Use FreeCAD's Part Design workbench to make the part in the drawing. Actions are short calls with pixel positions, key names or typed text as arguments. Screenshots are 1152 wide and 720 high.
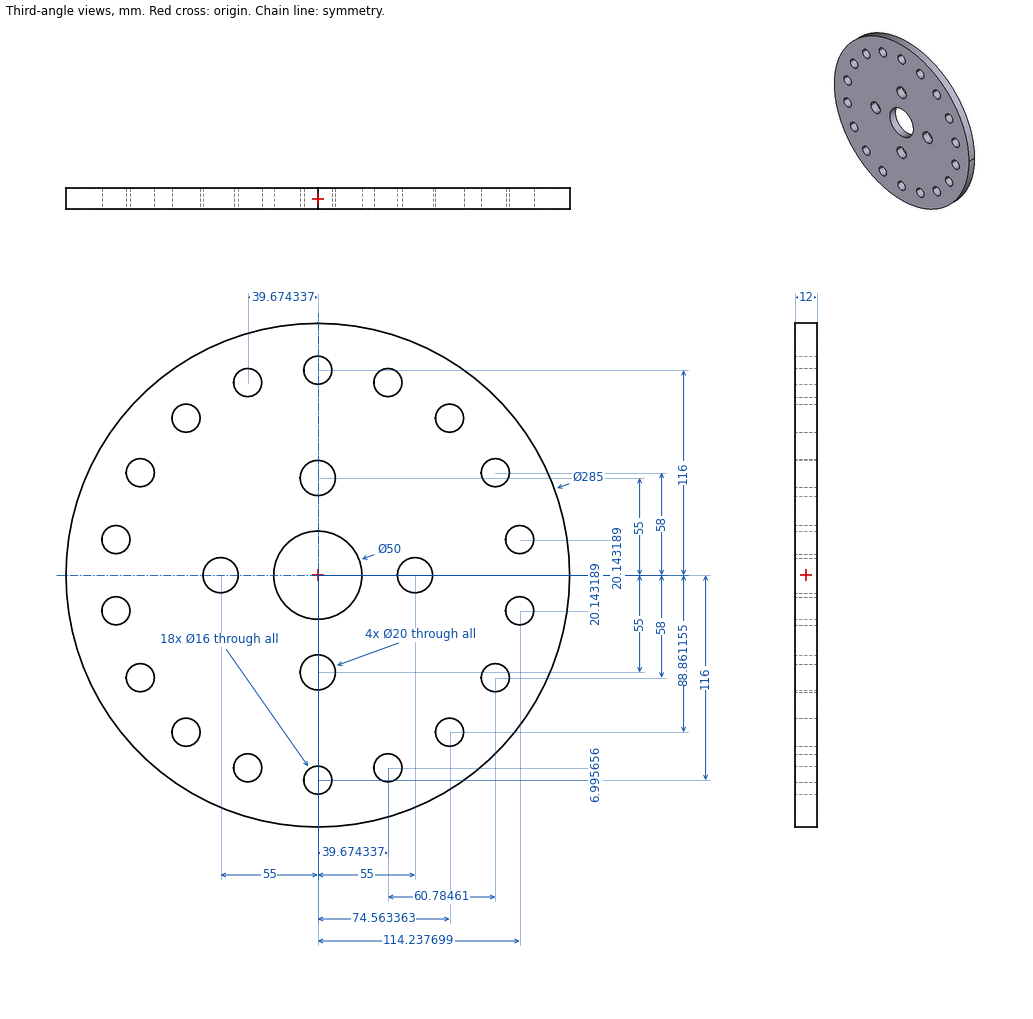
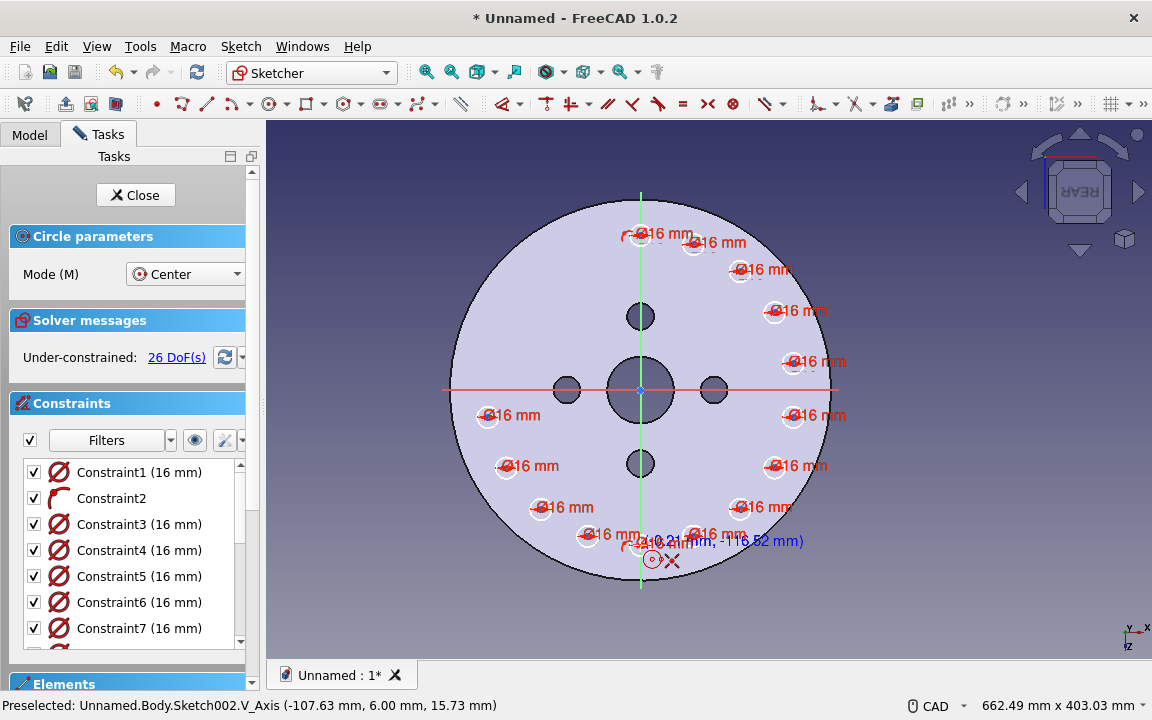
scroll(488, 363, up, 4)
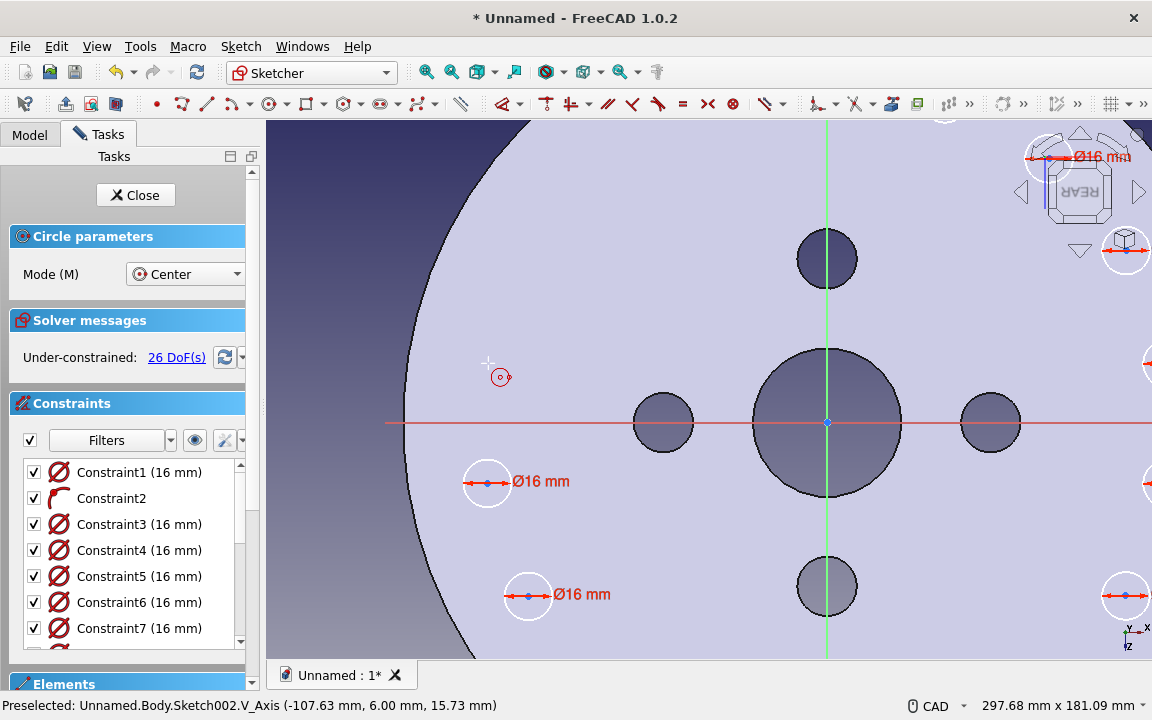
click(487, 363)
move(504, 346)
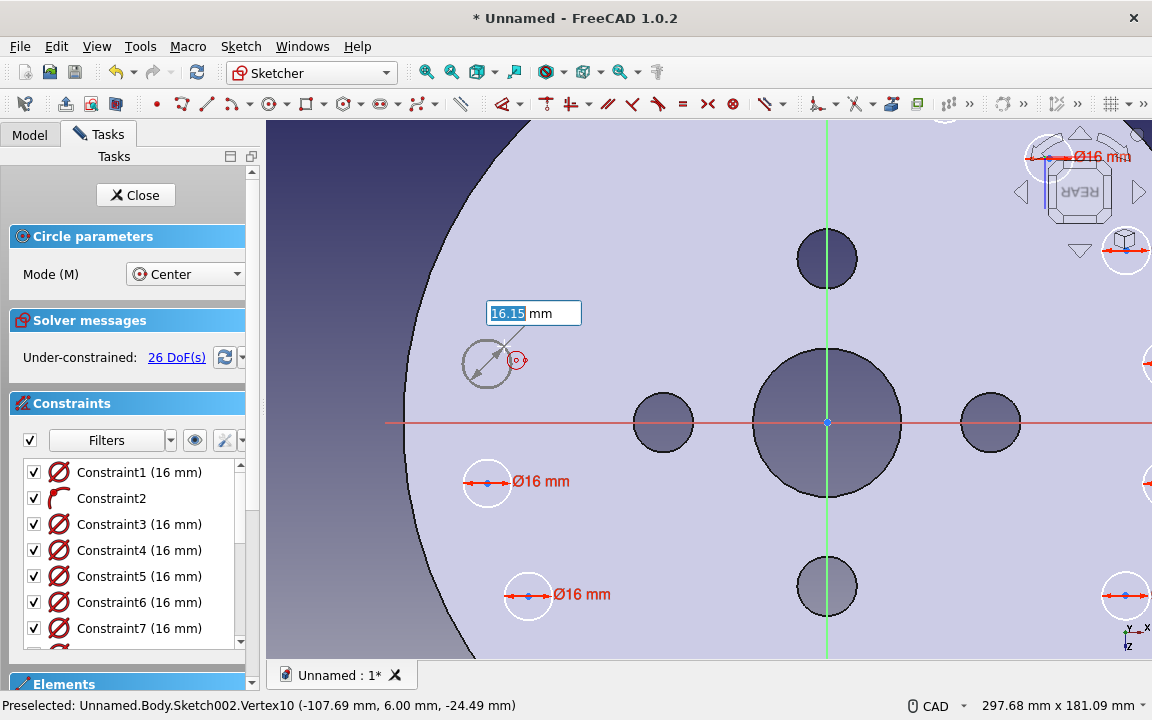
text(16)
key(Return)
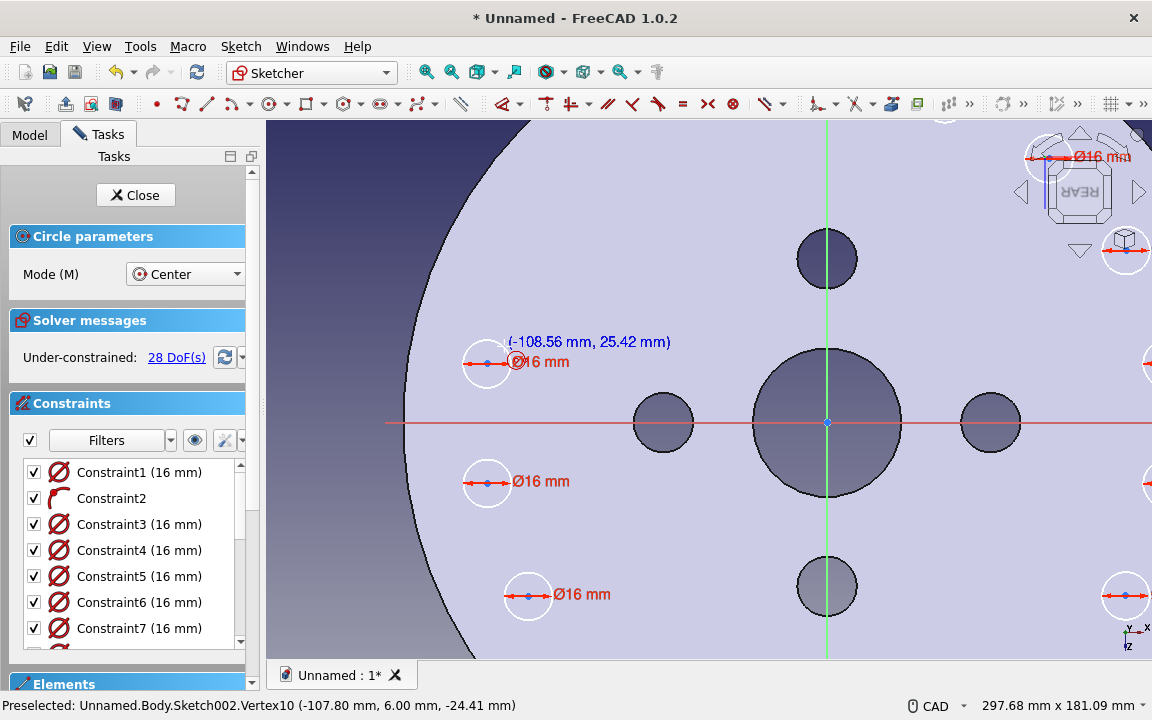
click(528, 250)
move(545, 233)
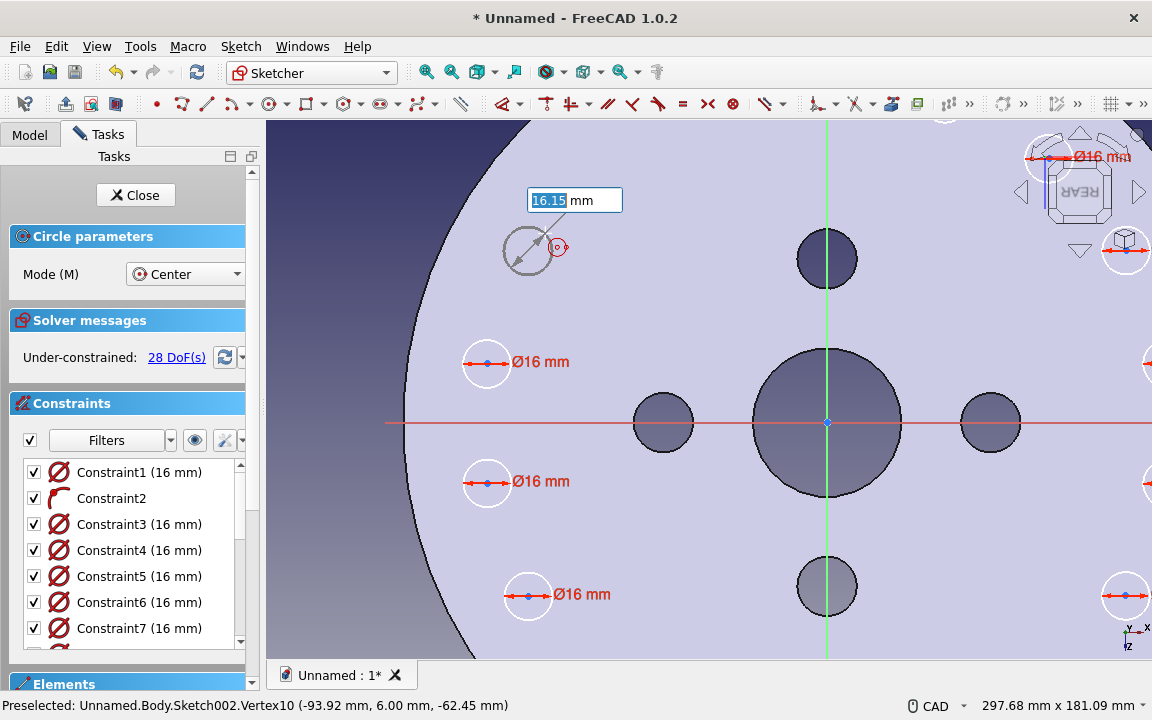
text(16)
key(Return)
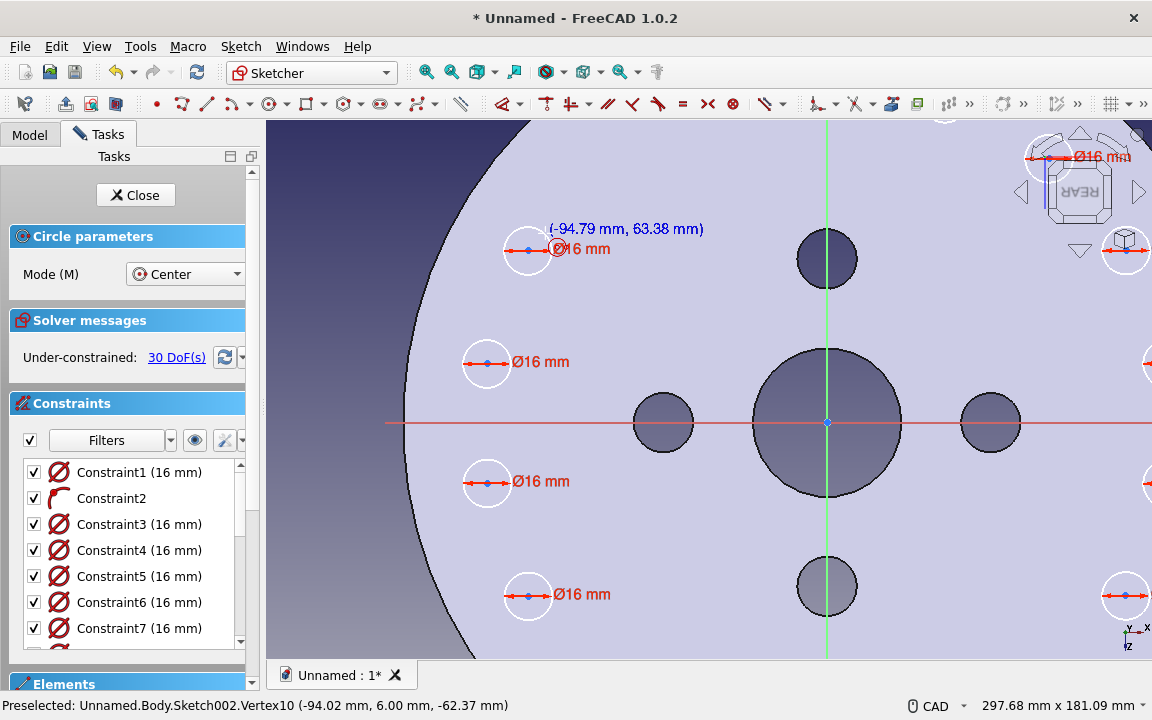
click(605, 158)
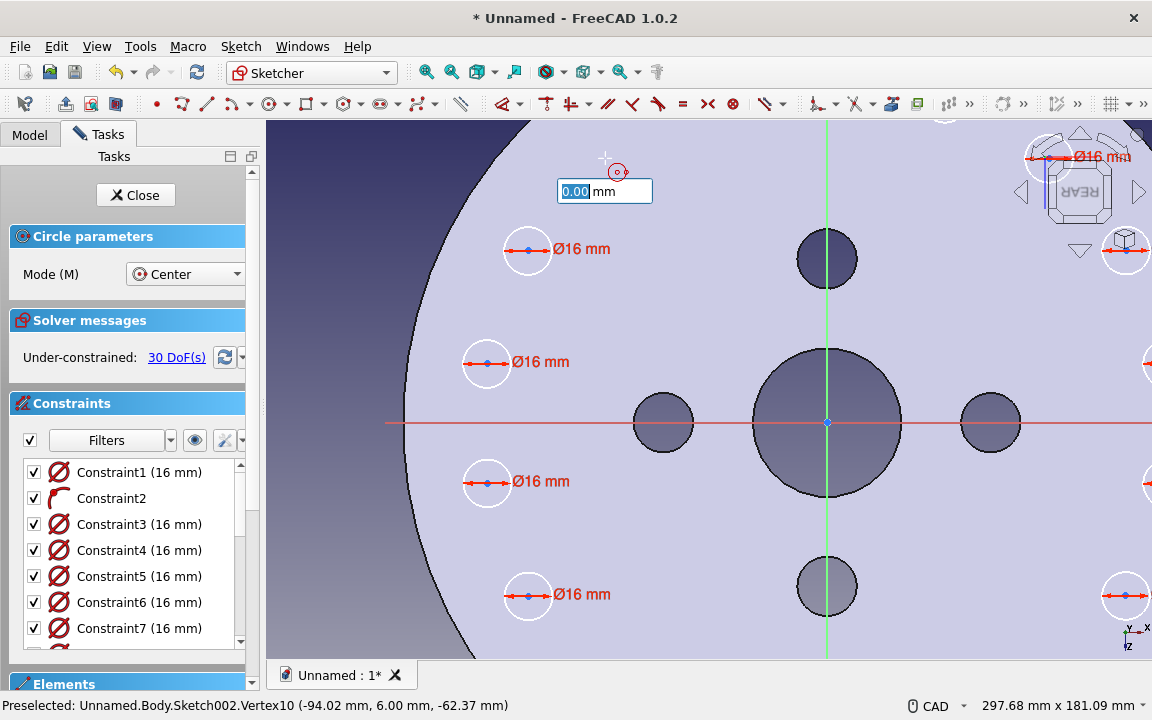
scroll(488, 362, down, 4)
move(548, 263)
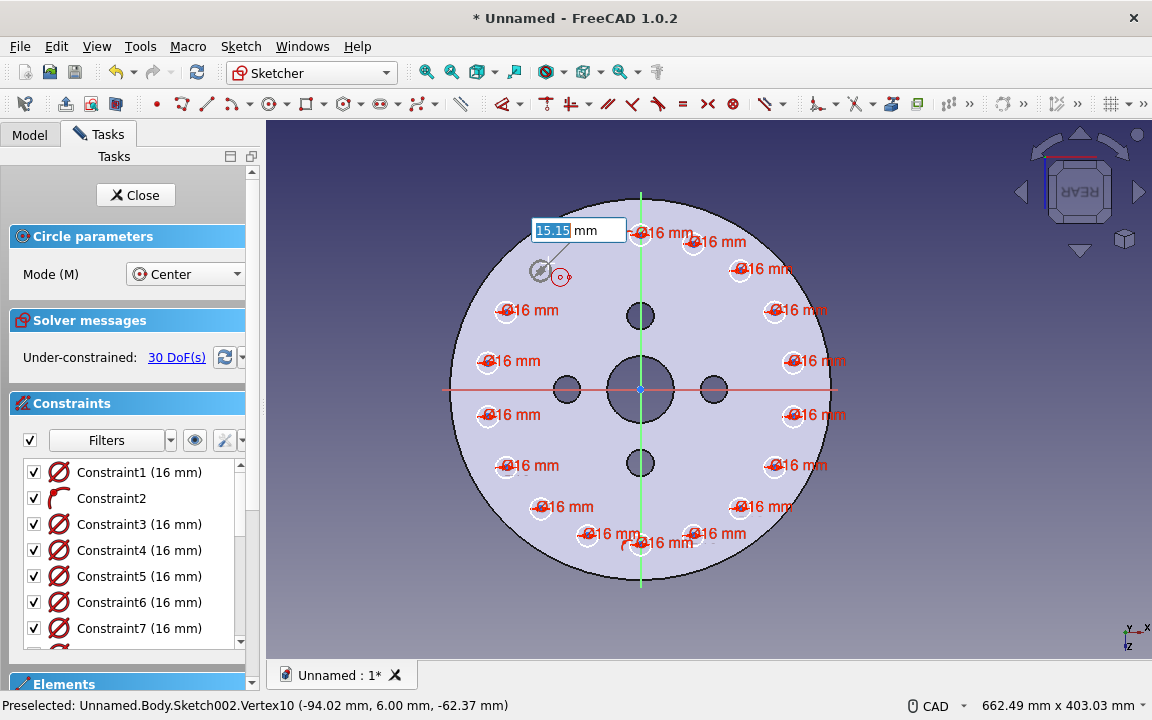
text(16)
key(Return)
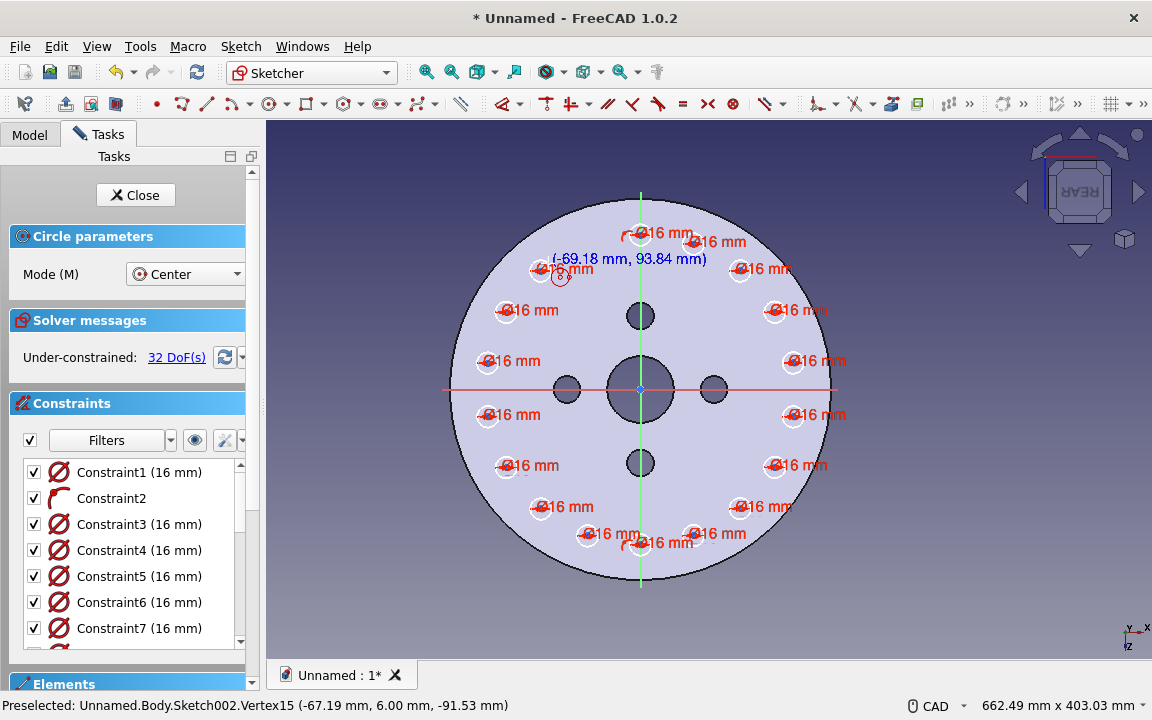
scroll(587, 244, up, 4)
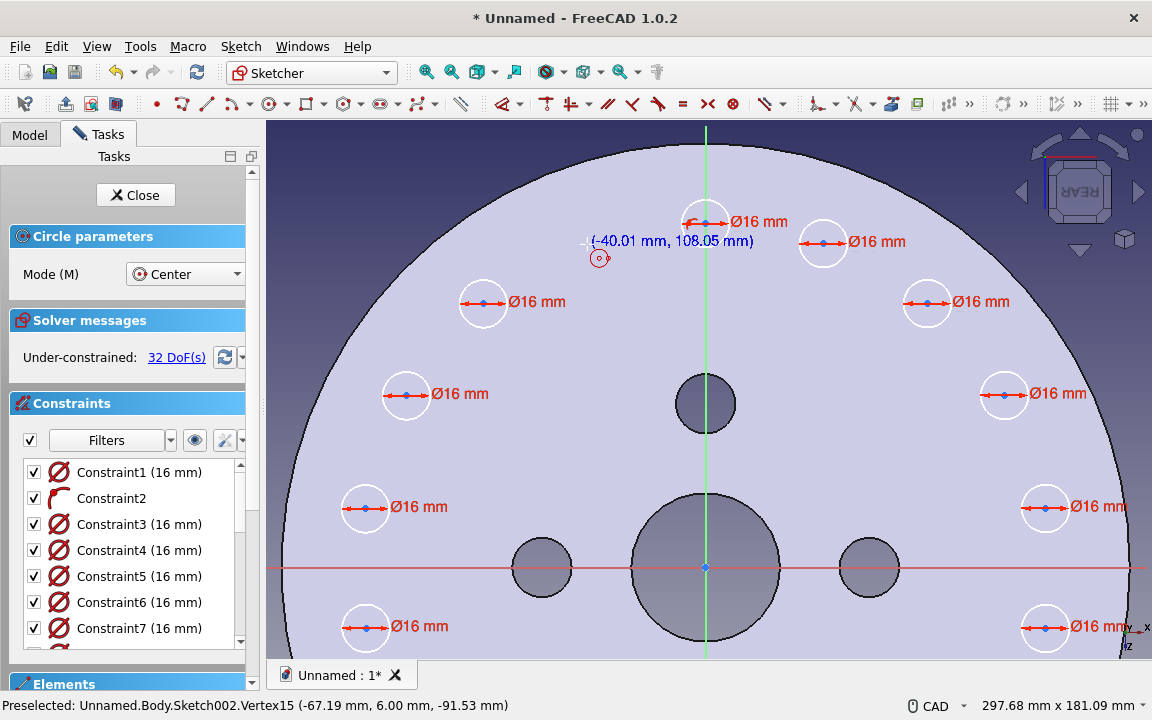
click(588, 243)
move(604, 226)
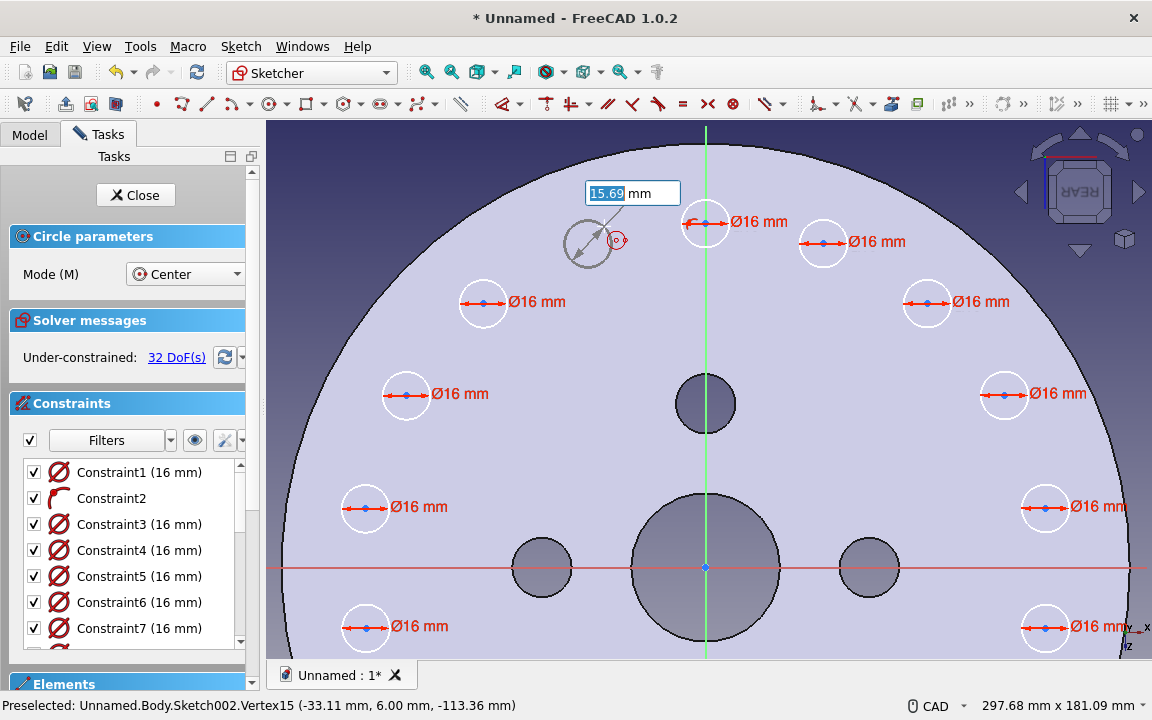
text(16)
key(Return)
key(Escape)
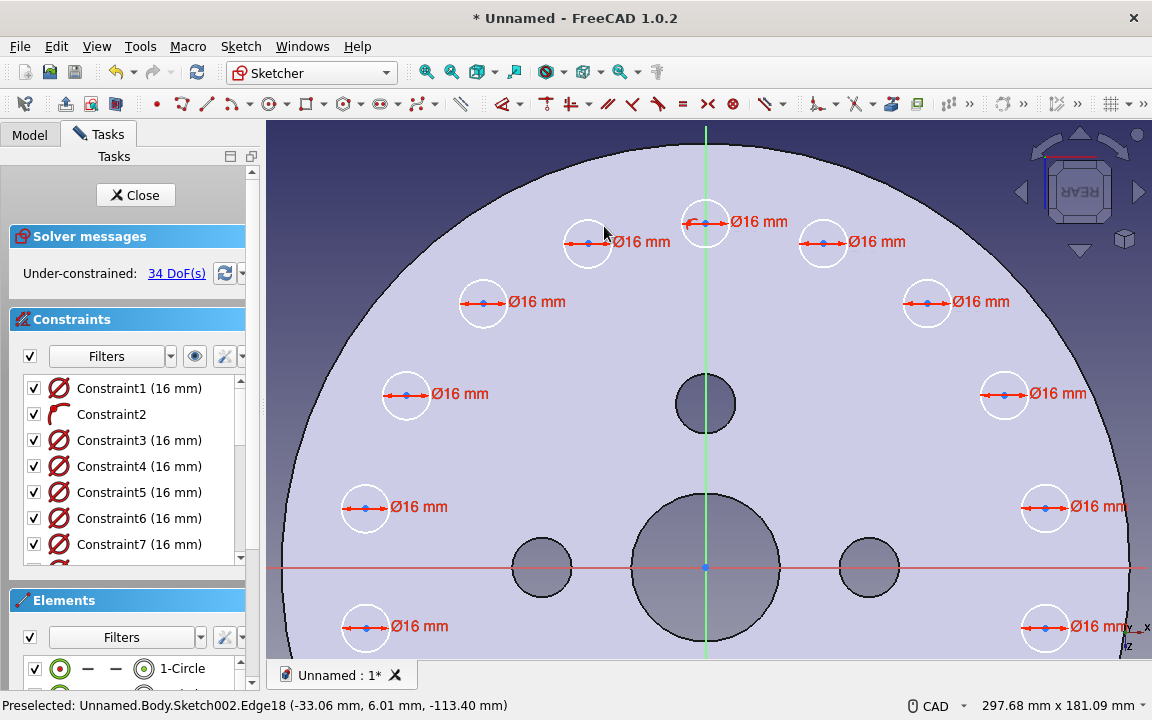
scroll(587, 244, down, 4)